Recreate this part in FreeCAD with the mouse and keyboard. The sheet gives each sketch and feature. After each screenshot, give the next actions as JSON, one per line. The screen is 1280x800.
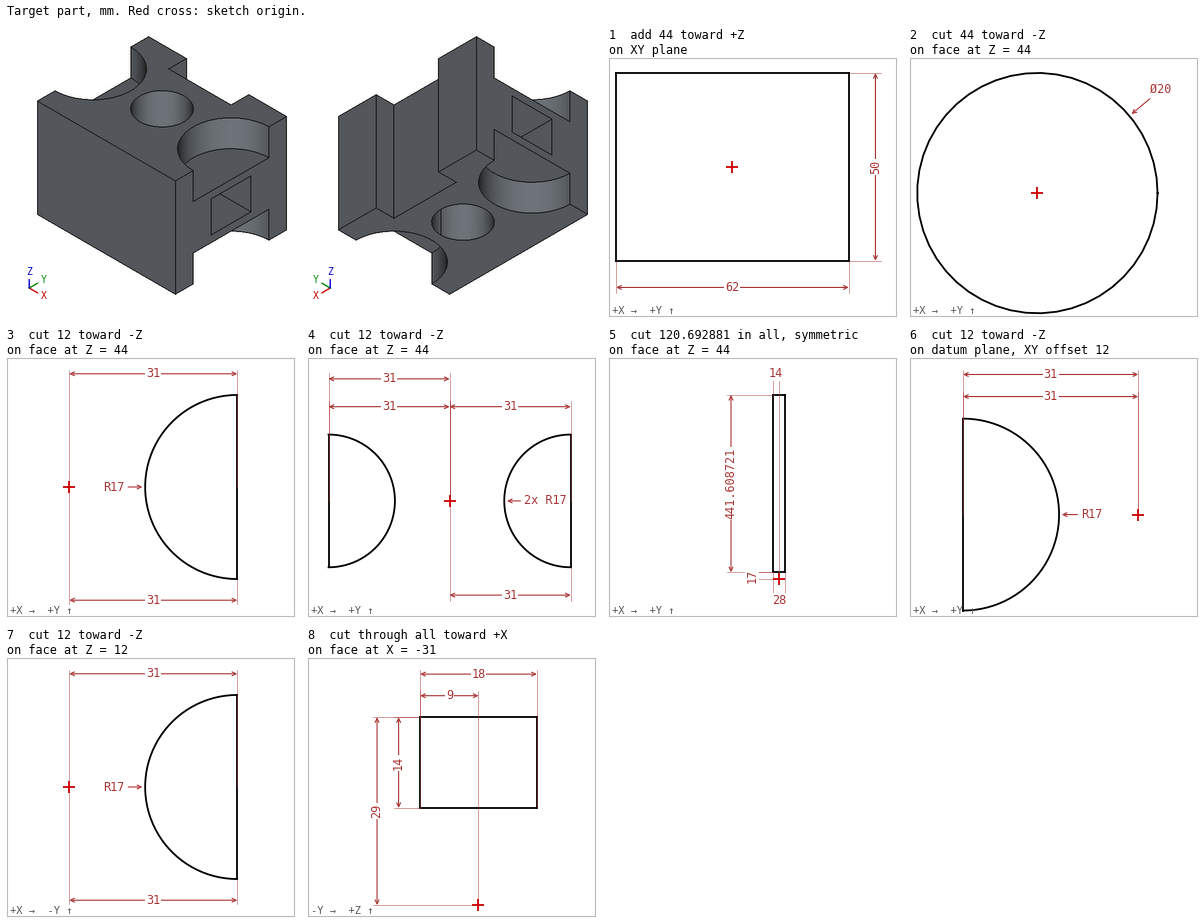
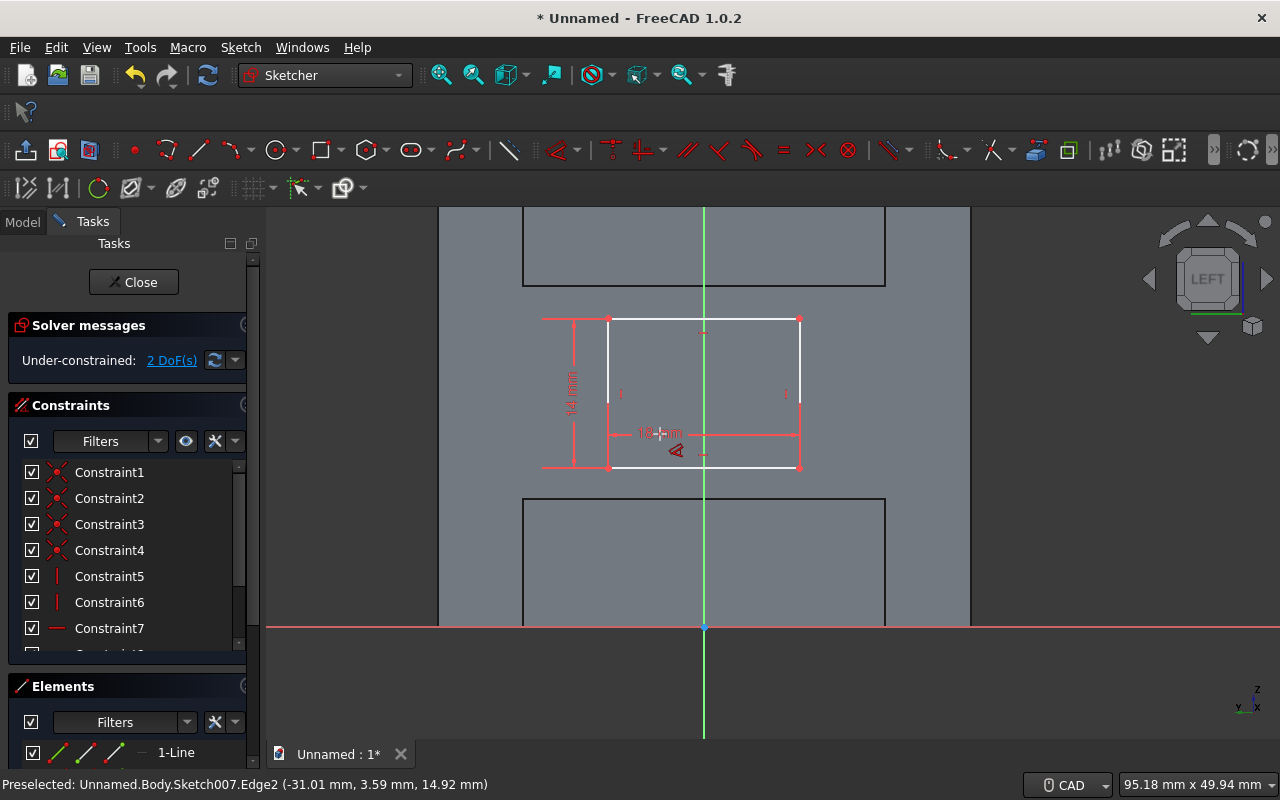
{"action": "left_click", "coordinate": [608, 319]}
{"action": "left_click", "coordinate": [656, 661]}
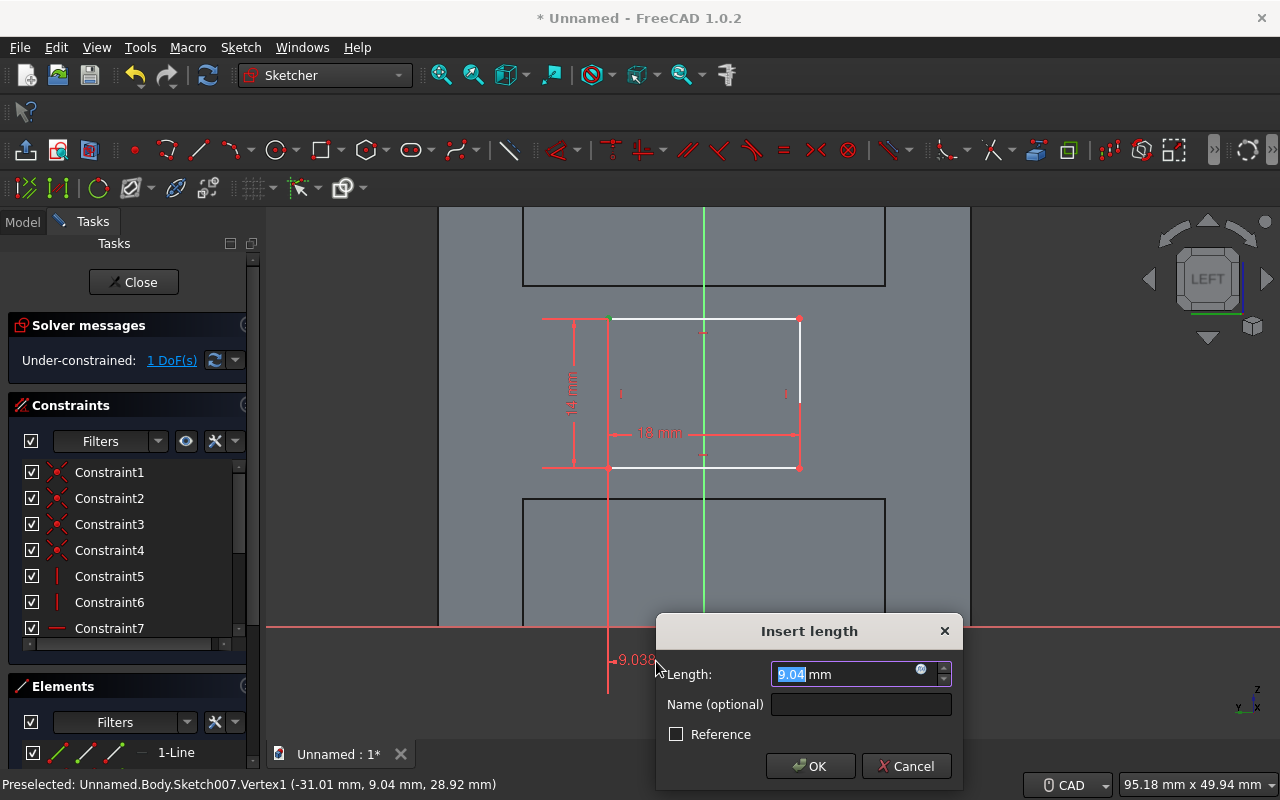
{"action": "type", "text": "9"}
{"action": "key", "text": "Return"}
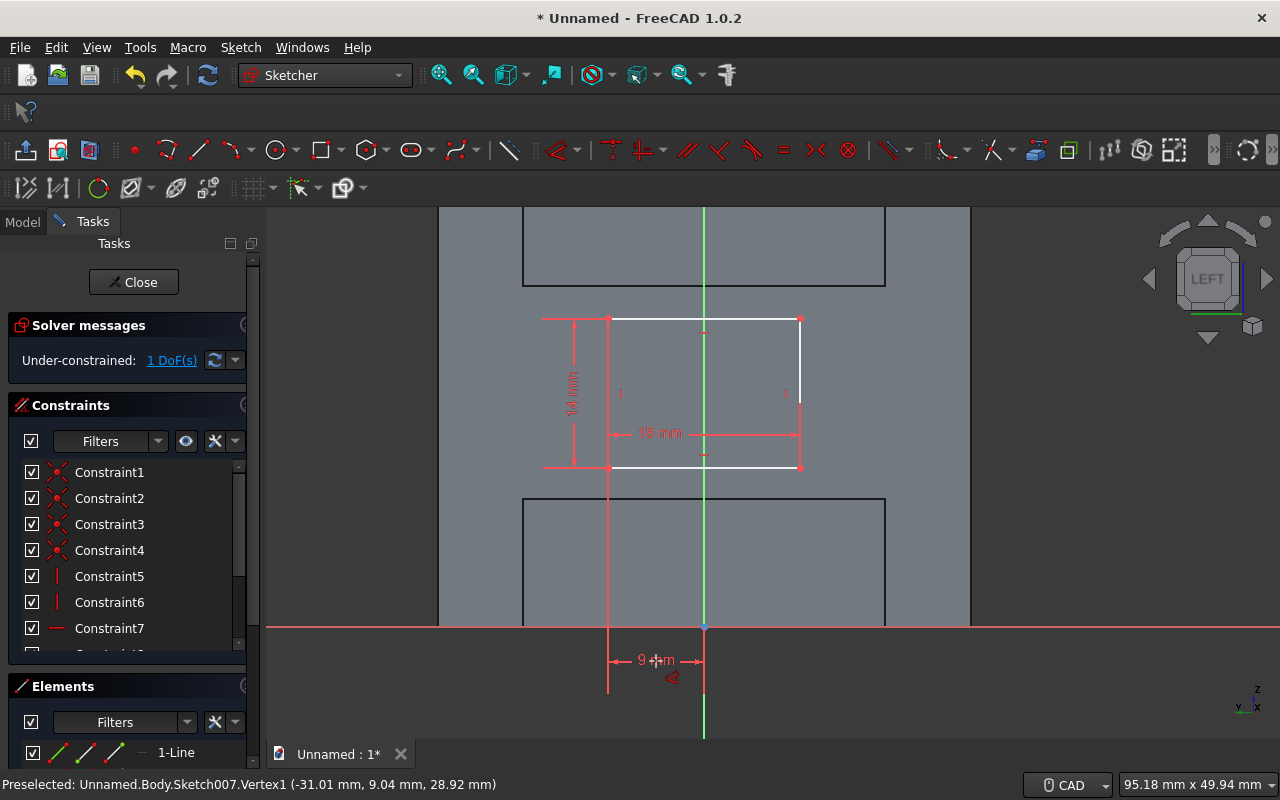
{"action": "left_click", "coordinate": [608, 319]}
{"action": "left_click", "coordinate": [574, 473]}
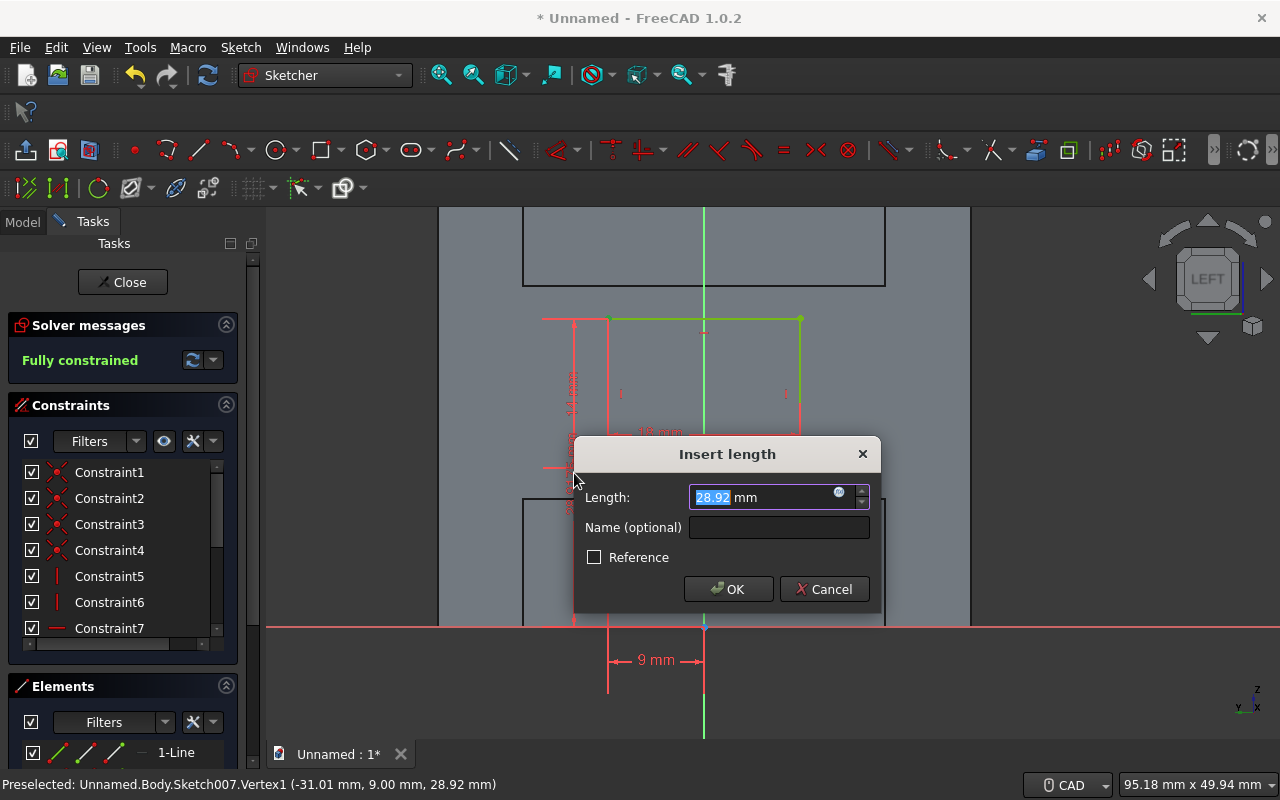
{"action": "type", "text": "29"}
{"action": "key", "text": "Return"}
{"action": "key", "text": "Escape"}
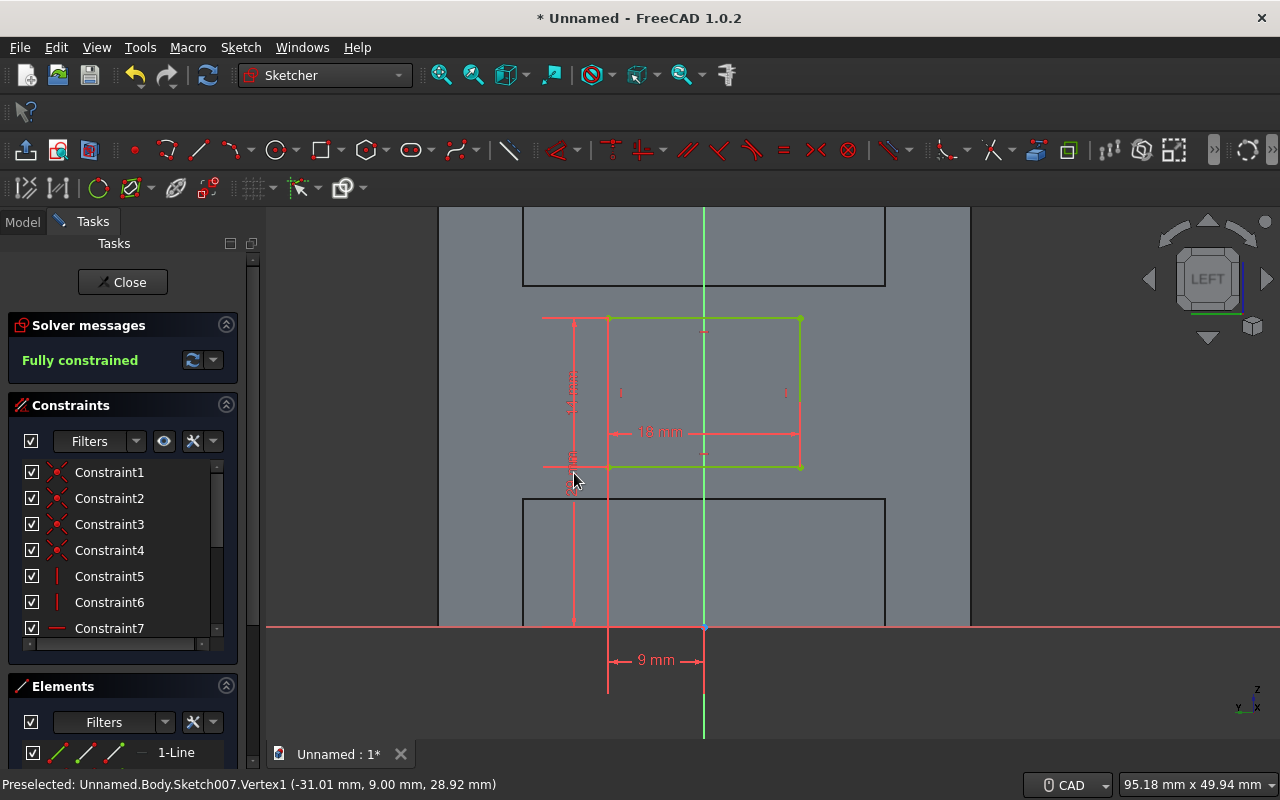
{"action": "left_click", "coordinate": [123, 282]}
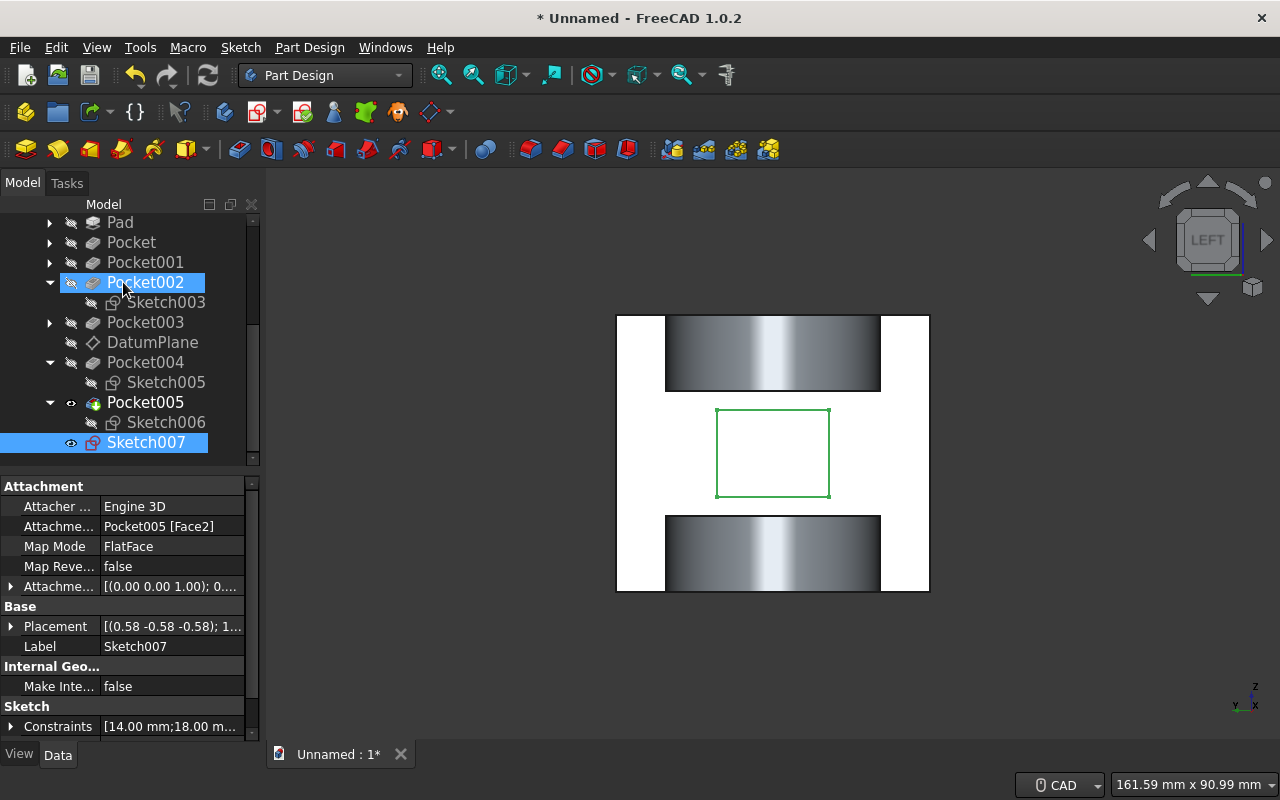
{"action": "left_click", "coordinate": [240, 150]}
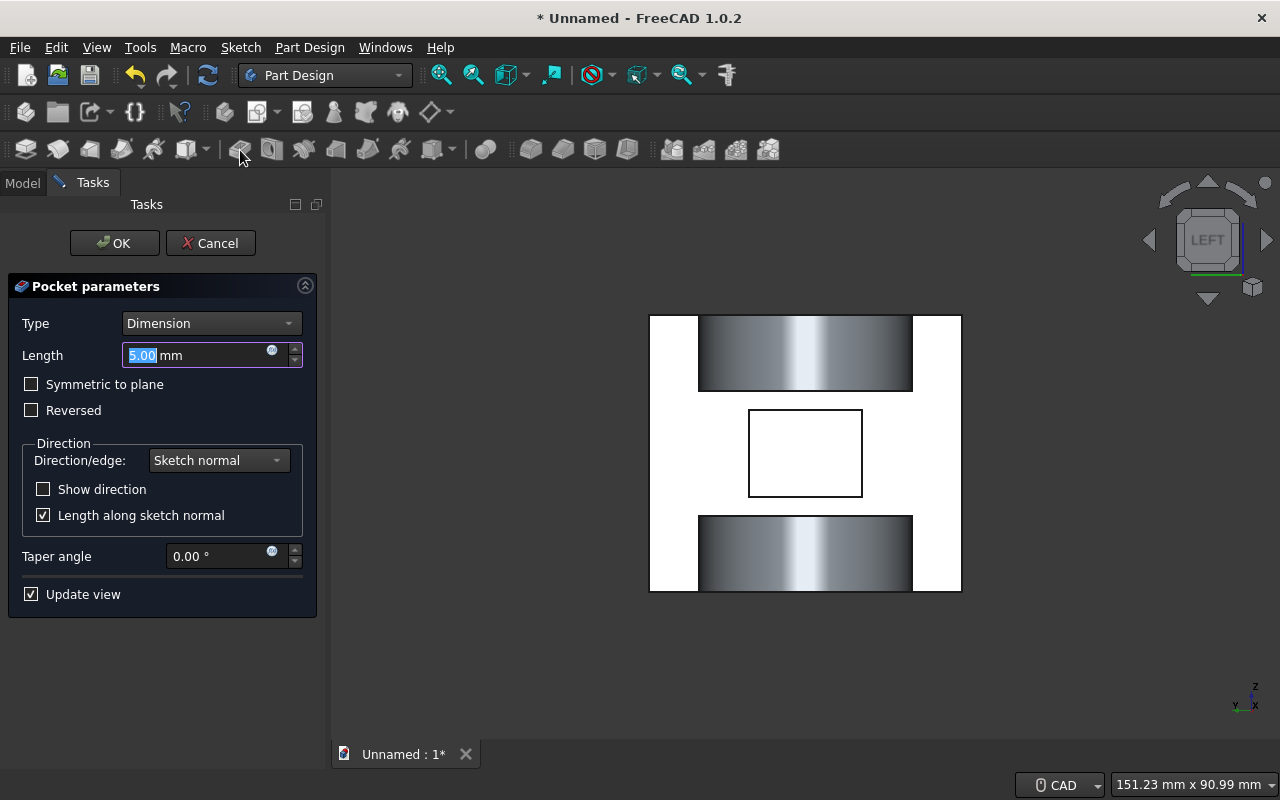
{"action": "left_click", "coordinate": [212, 324]}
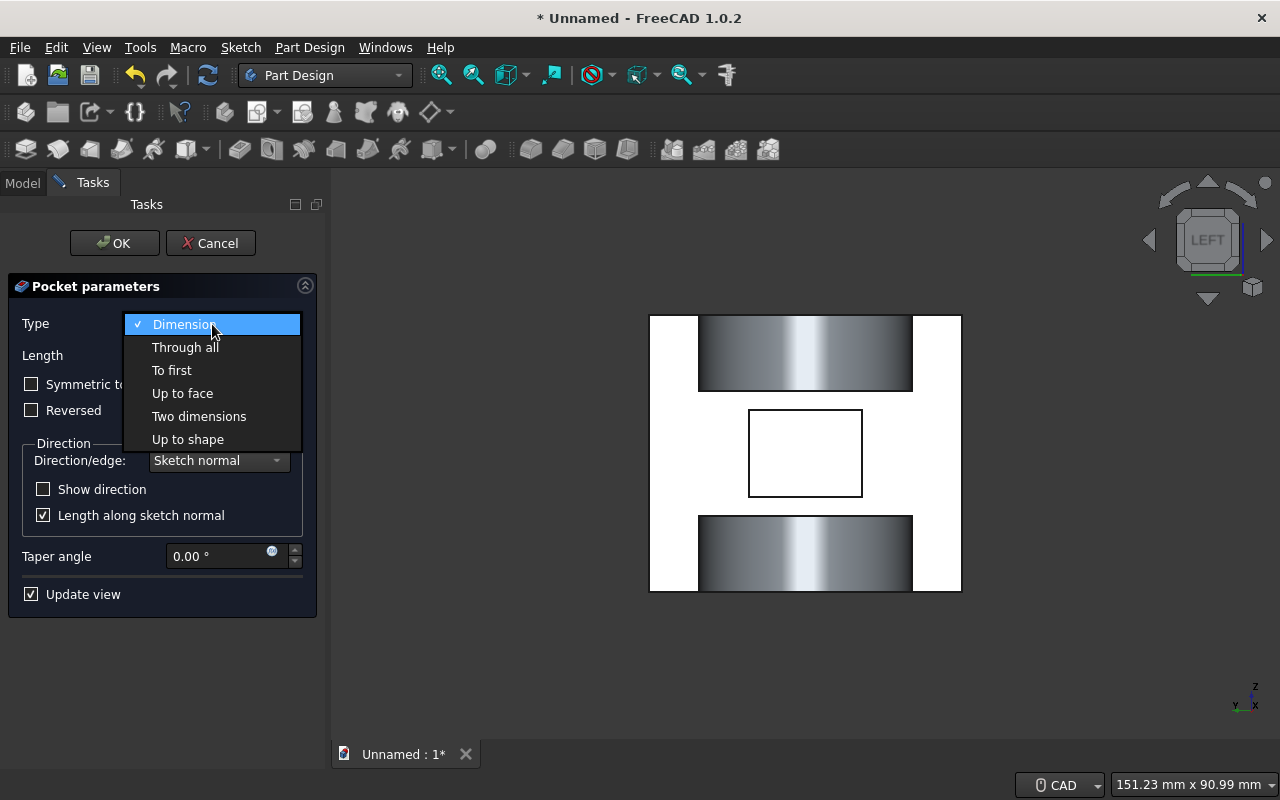
{"action": "left_click", "coordinate": [212, 348]}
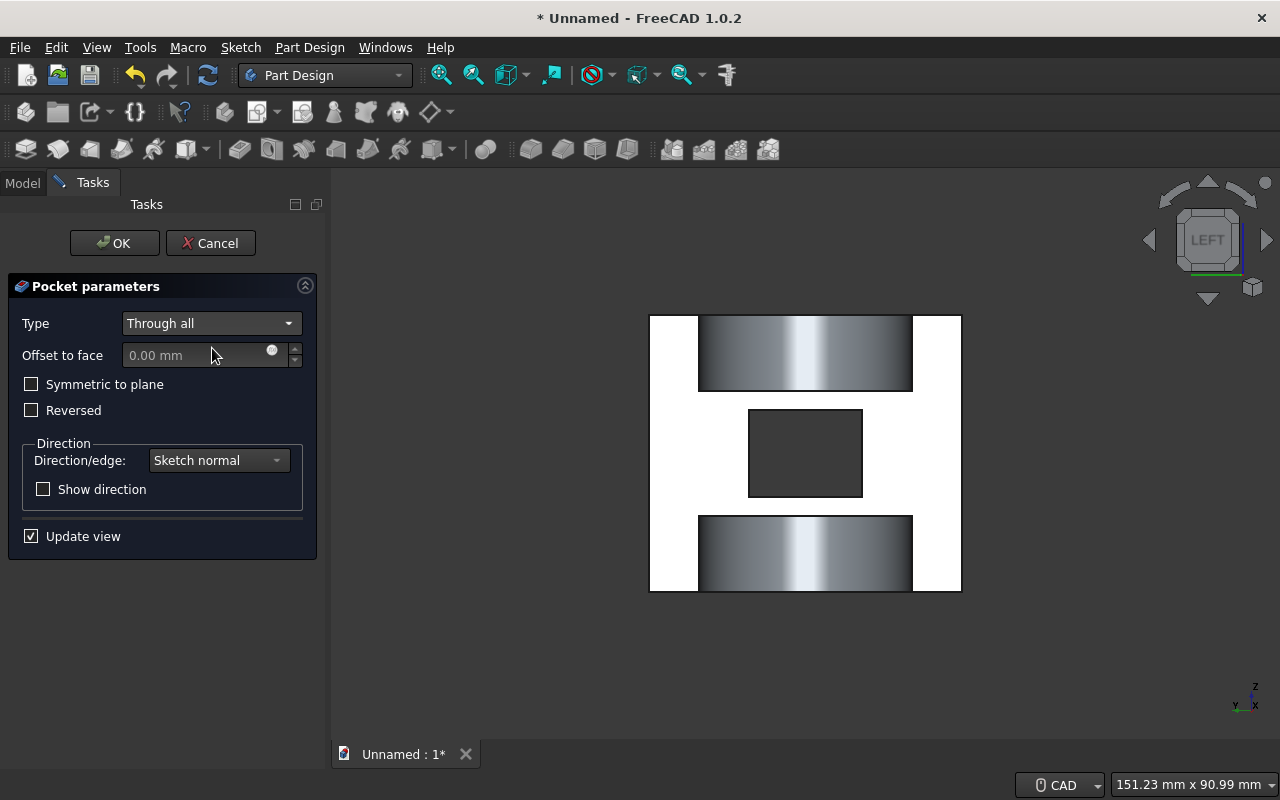
{"action": "left_click", "coordinate": [115, 243]}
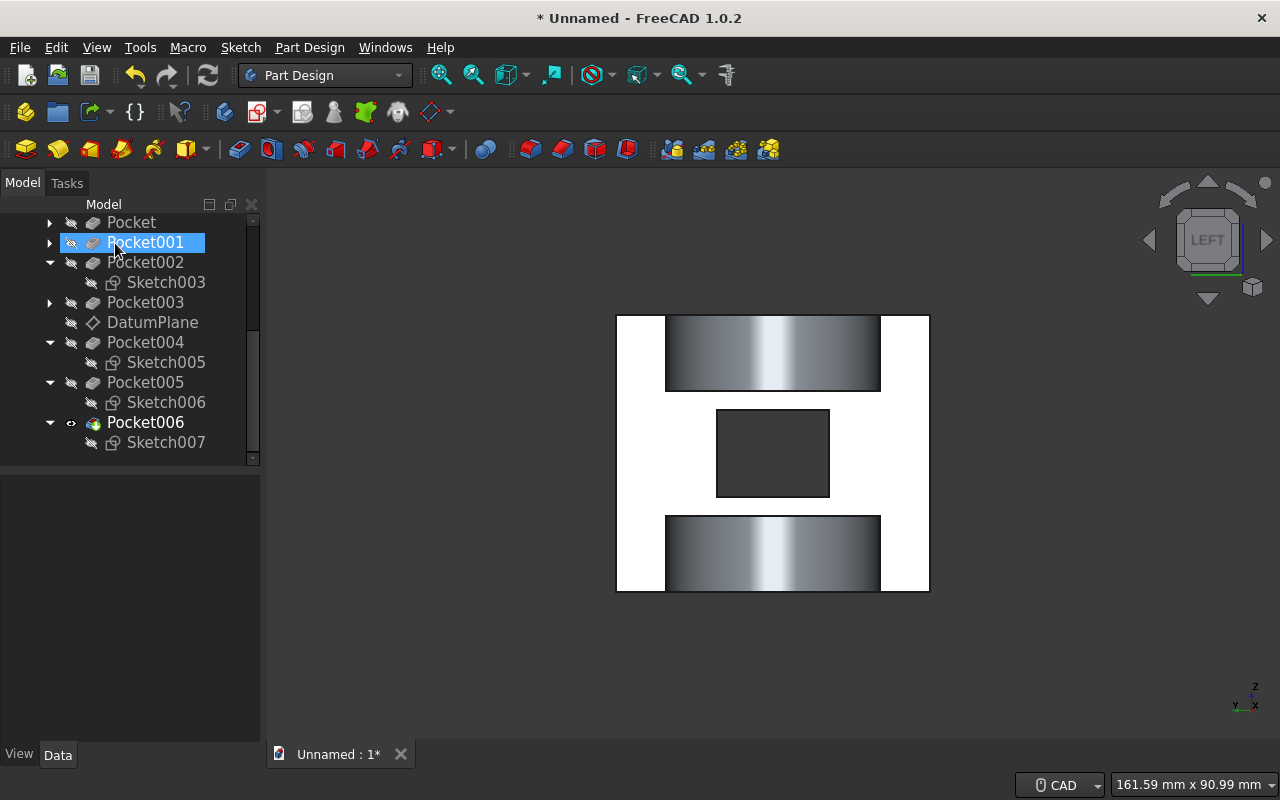
{"action": "key", "text": "0"}